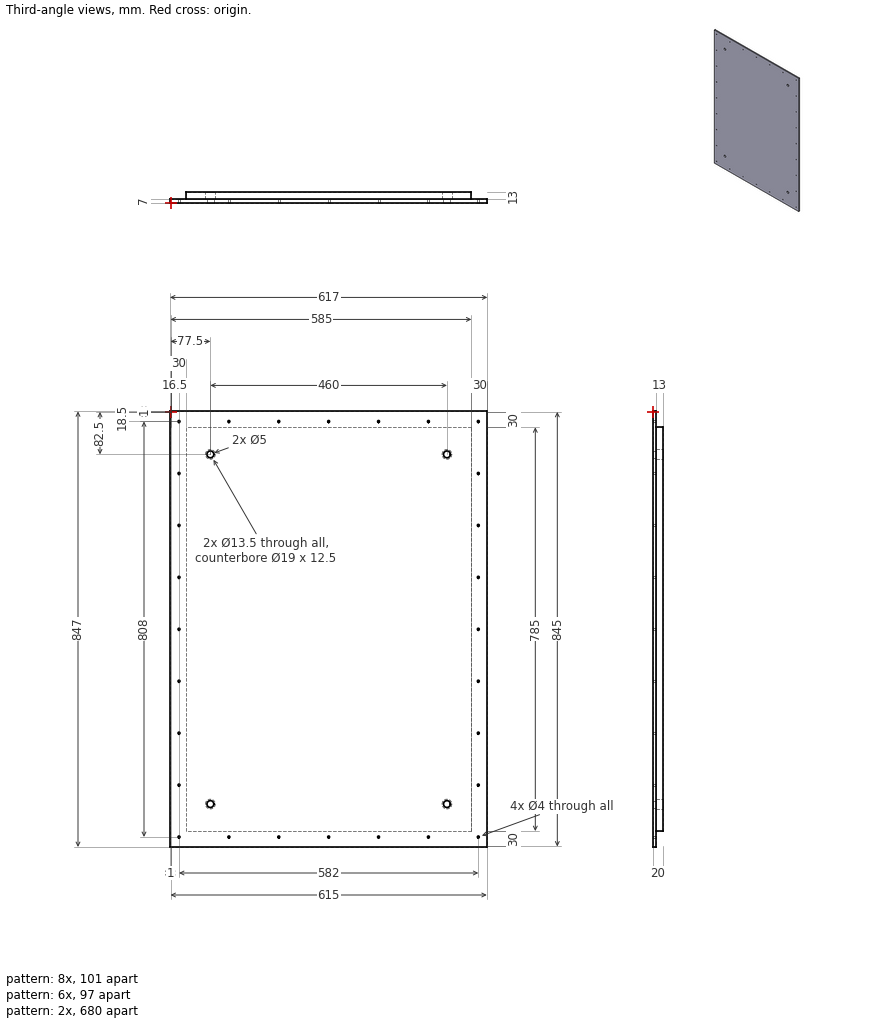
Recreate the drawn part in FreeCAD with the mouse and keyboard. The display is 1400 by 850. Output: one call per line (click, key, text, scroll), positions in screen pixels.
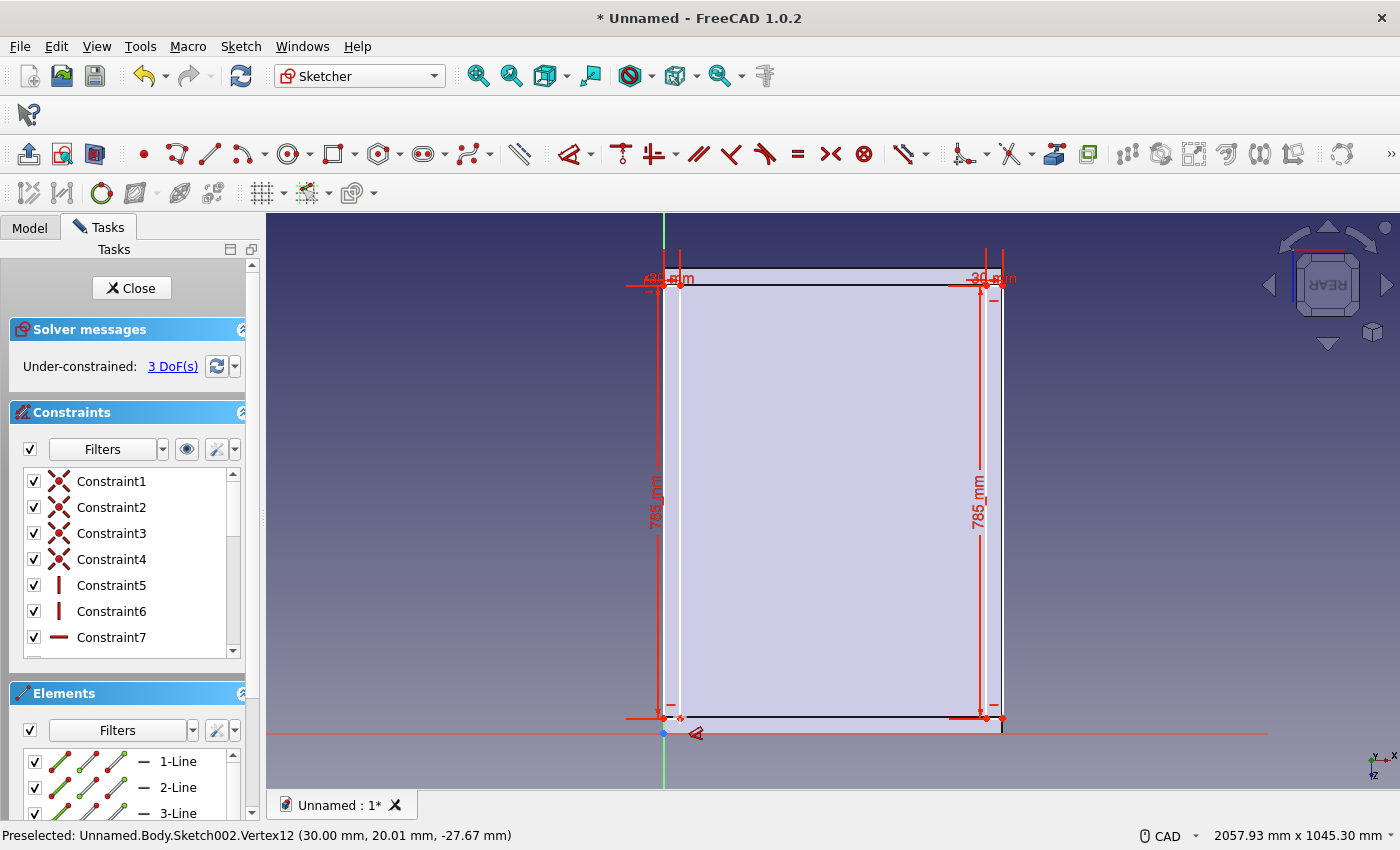
scroll(986, 719, up, 5)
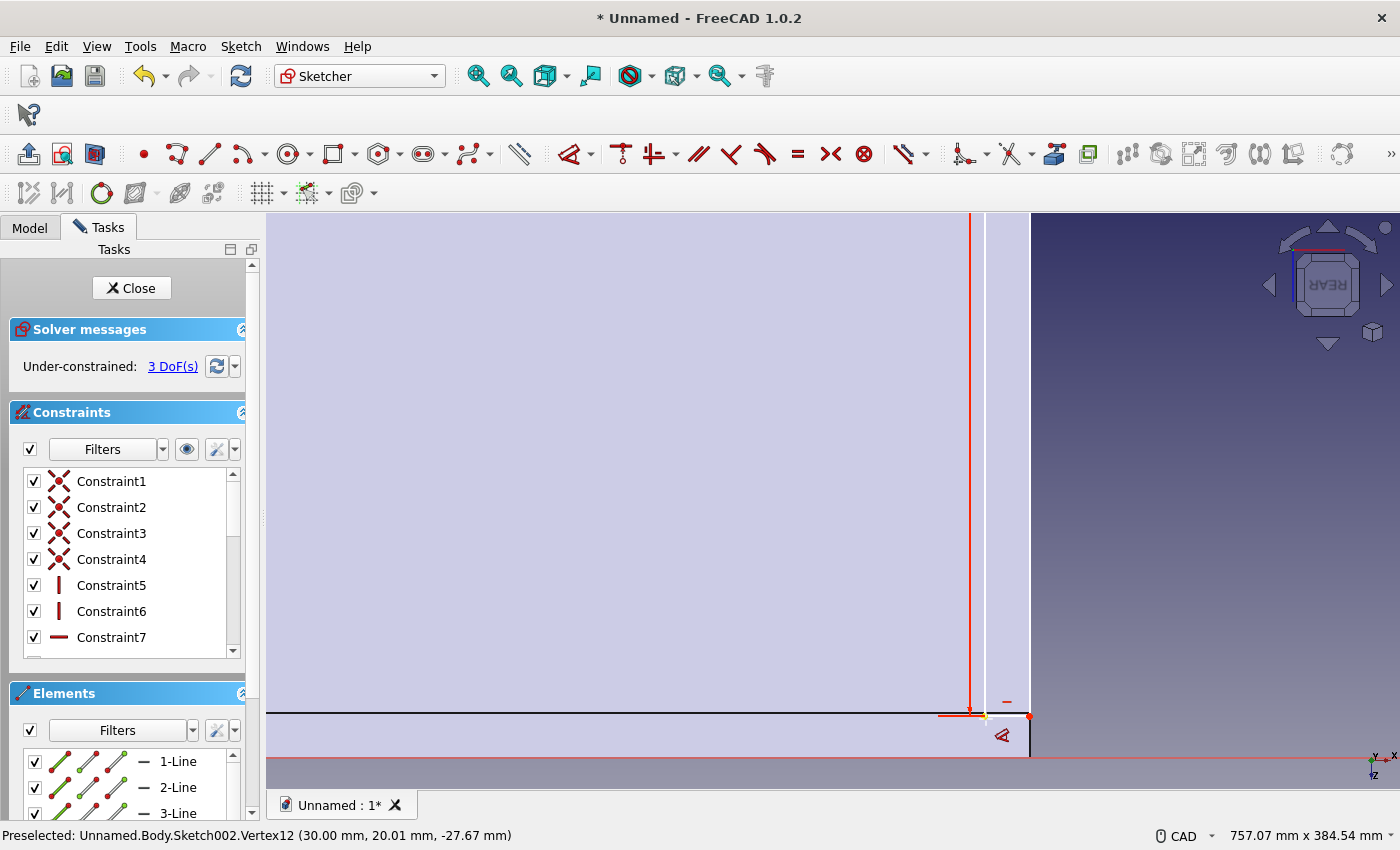
click(985, 716)
click(1019, 737)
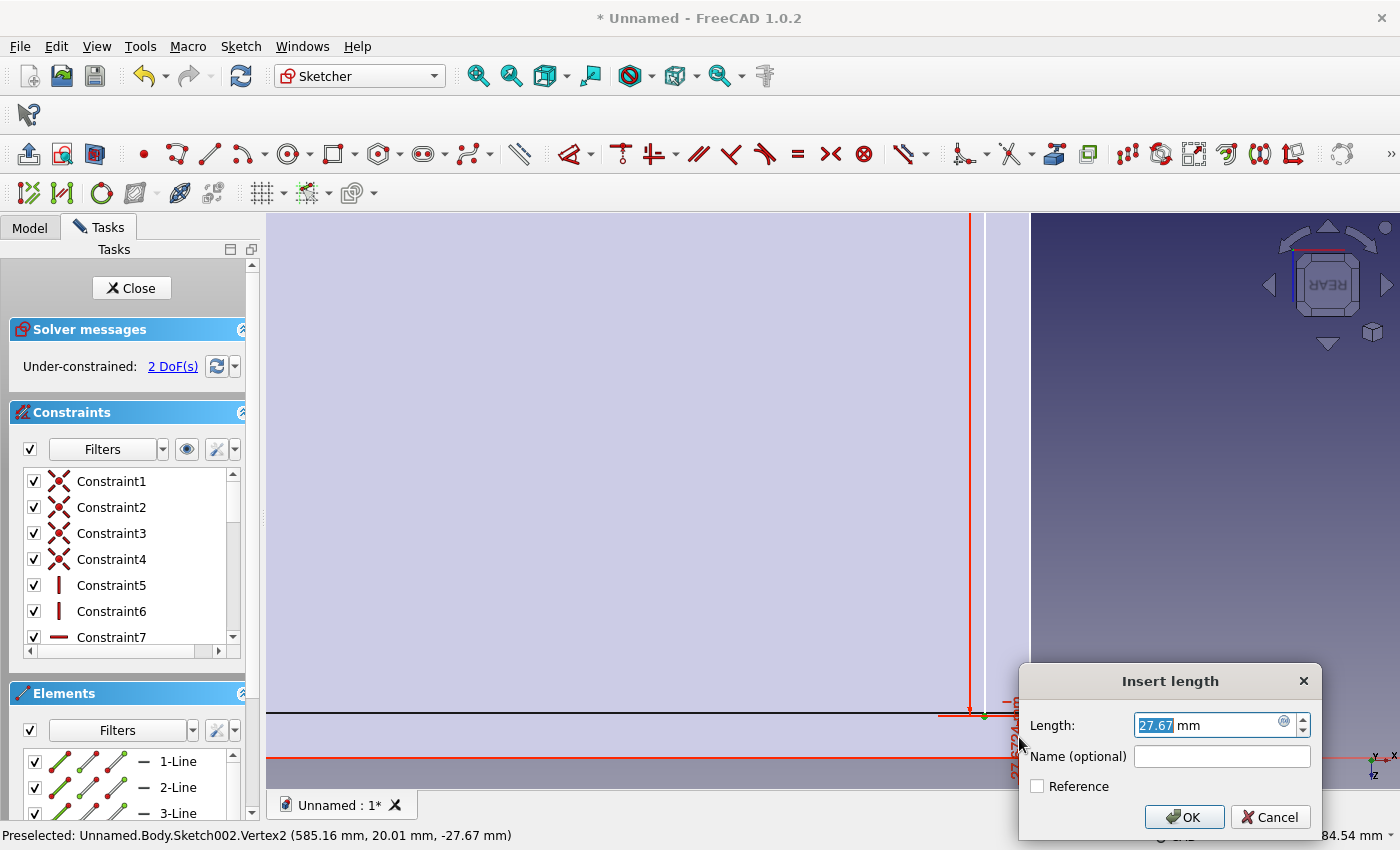
text(30)
key(Return)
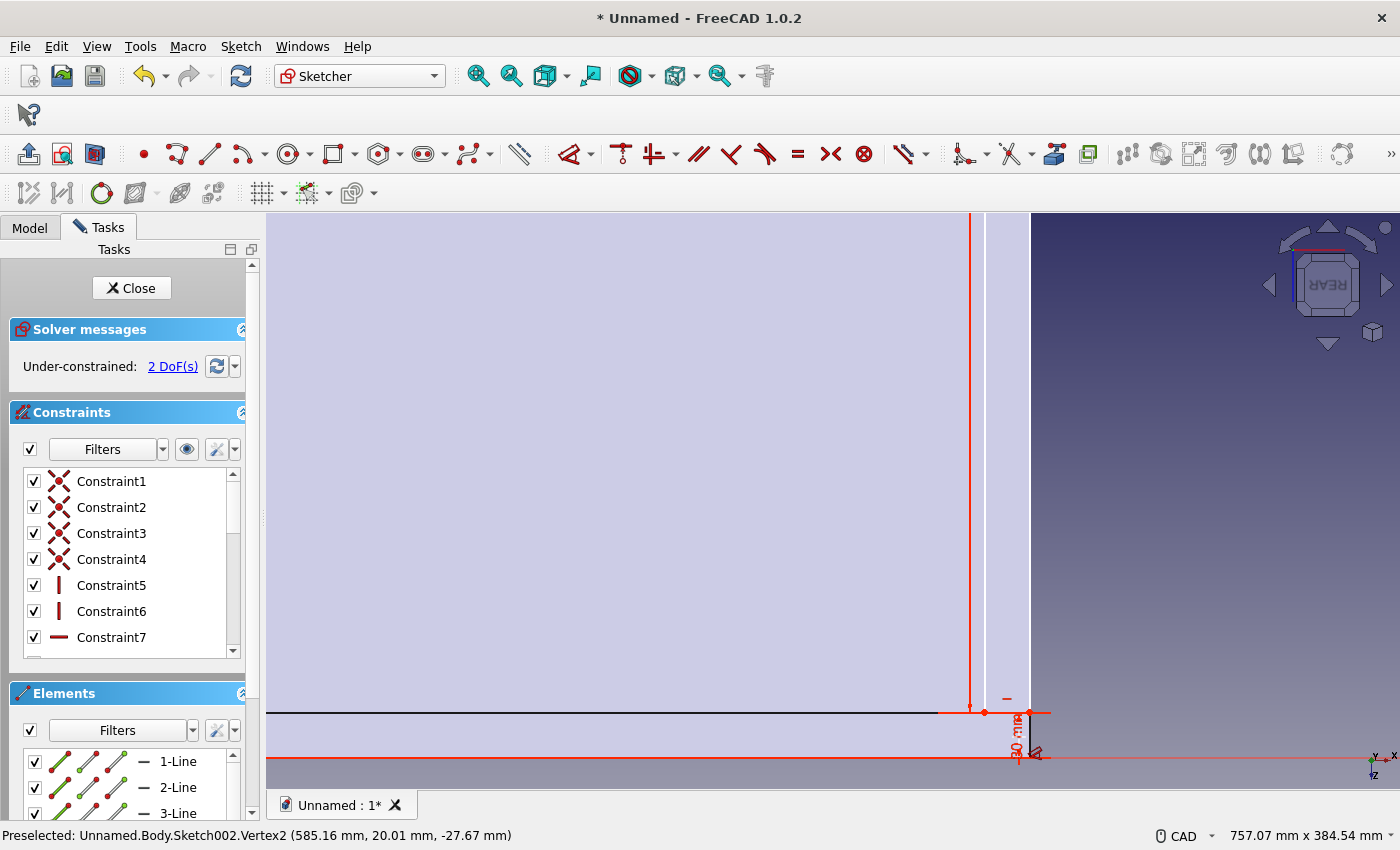
scroll(849, 653, down, 6)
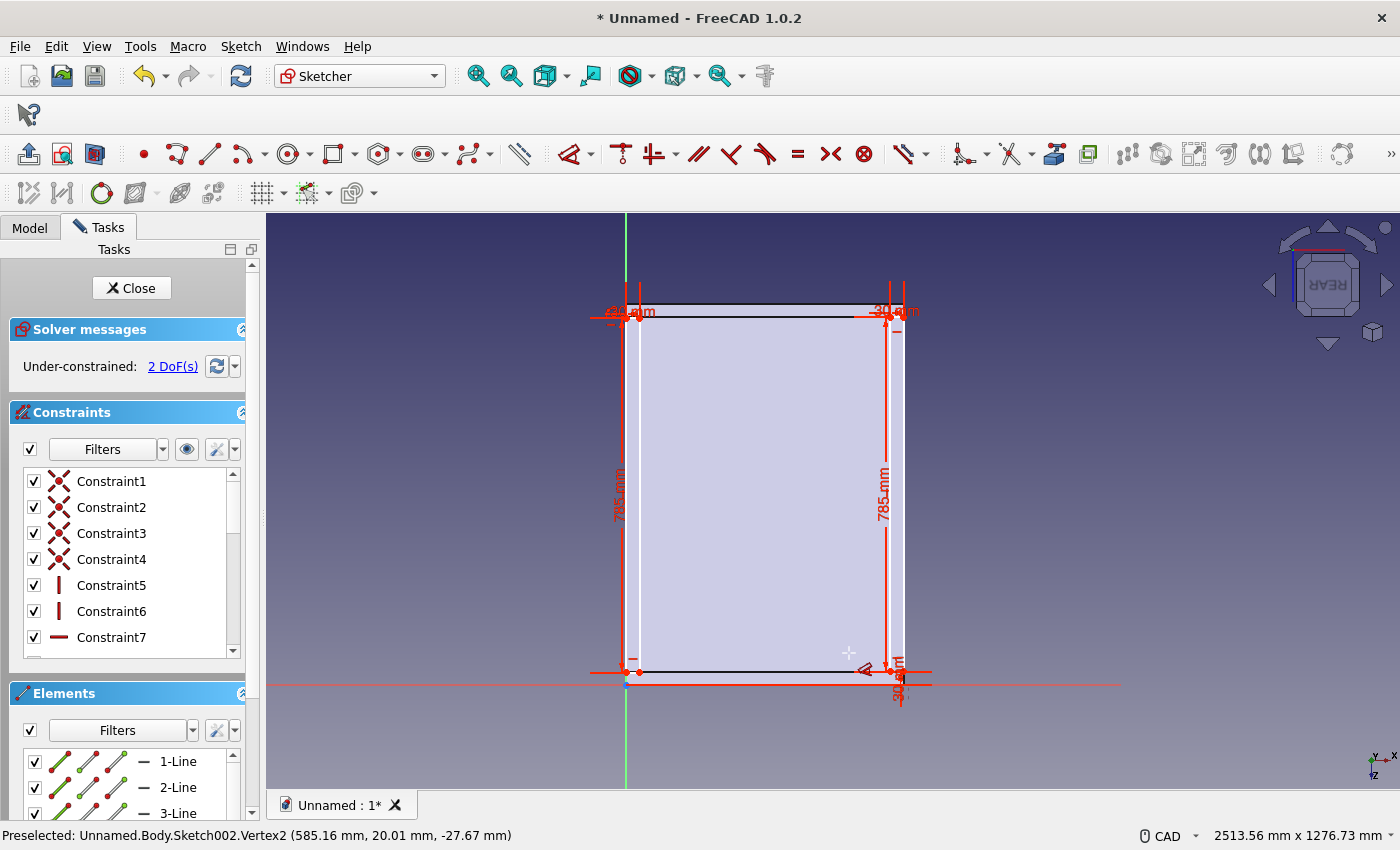
scroll(626, 673, up, 6)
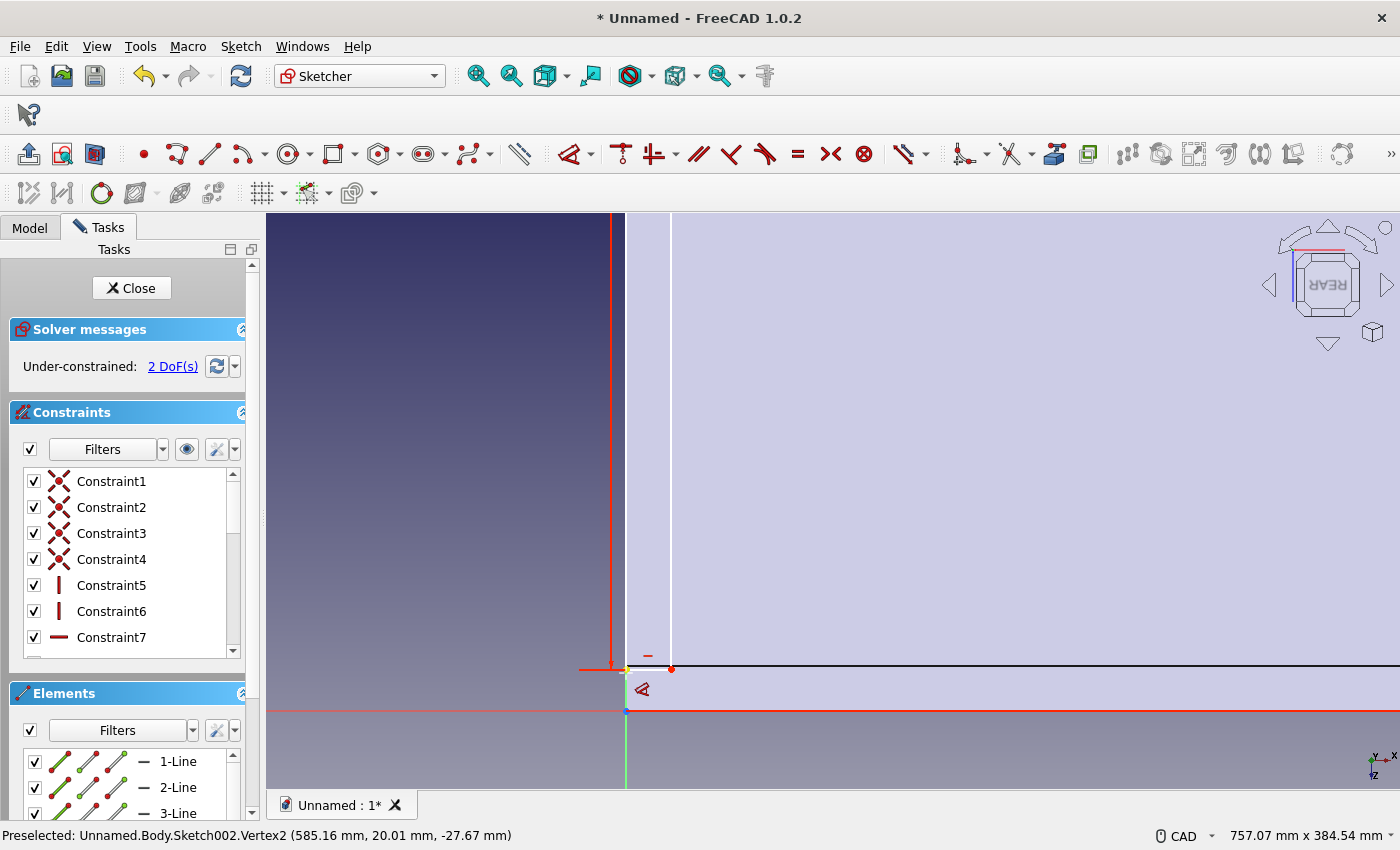
click(626, 670)
click(592, 691)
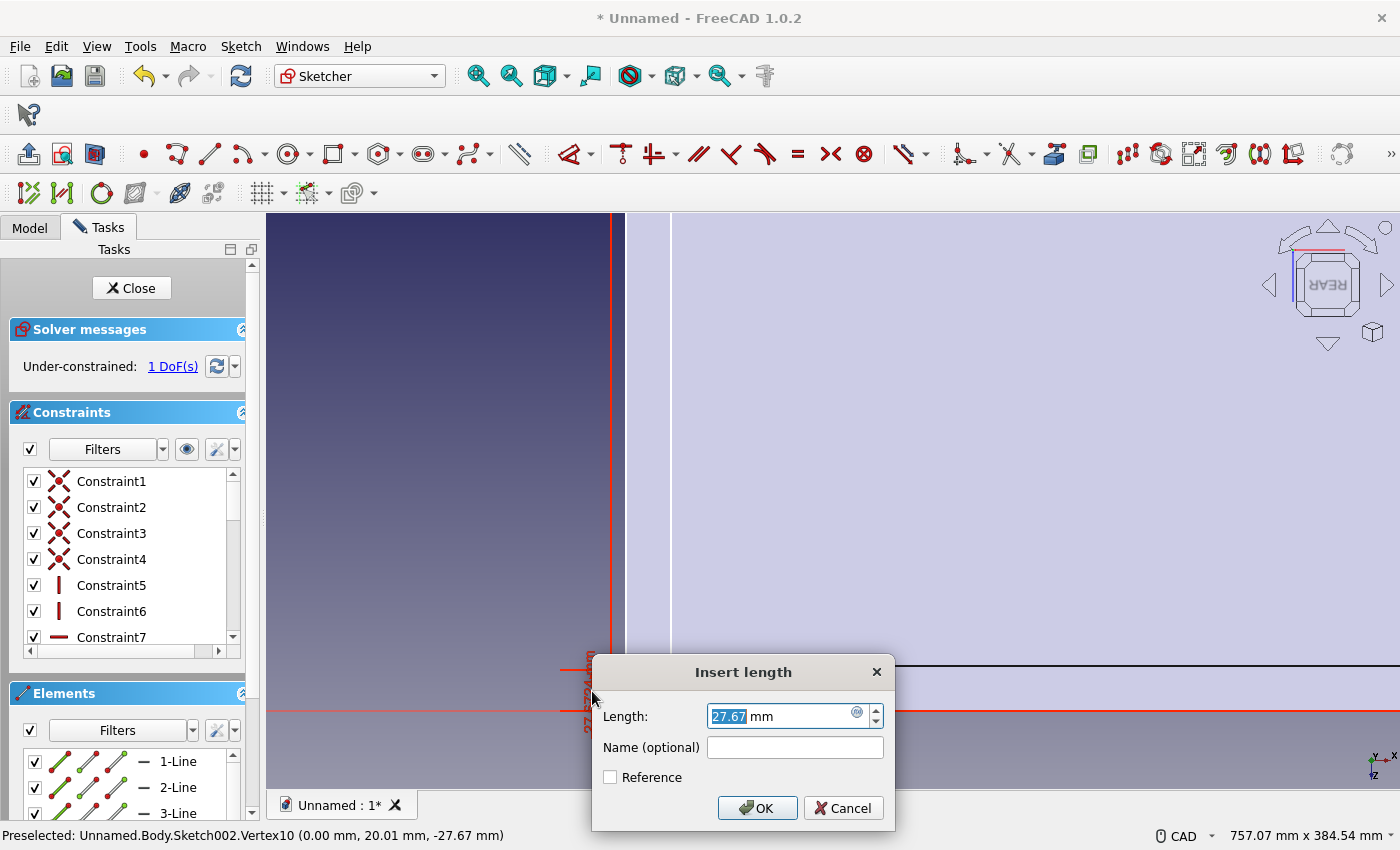
text(30)
key(Return)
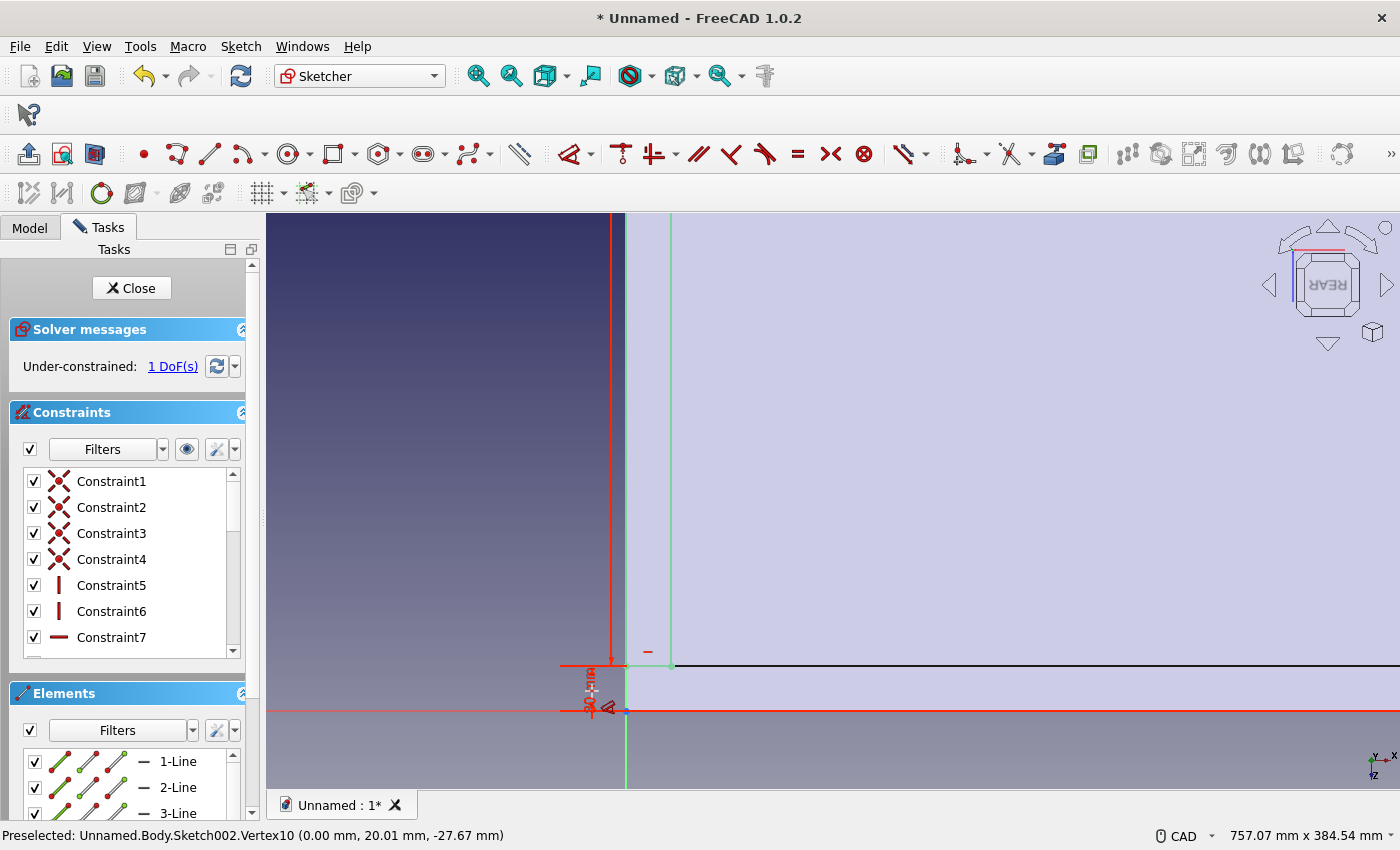
scroll(626, 673, down, 6)